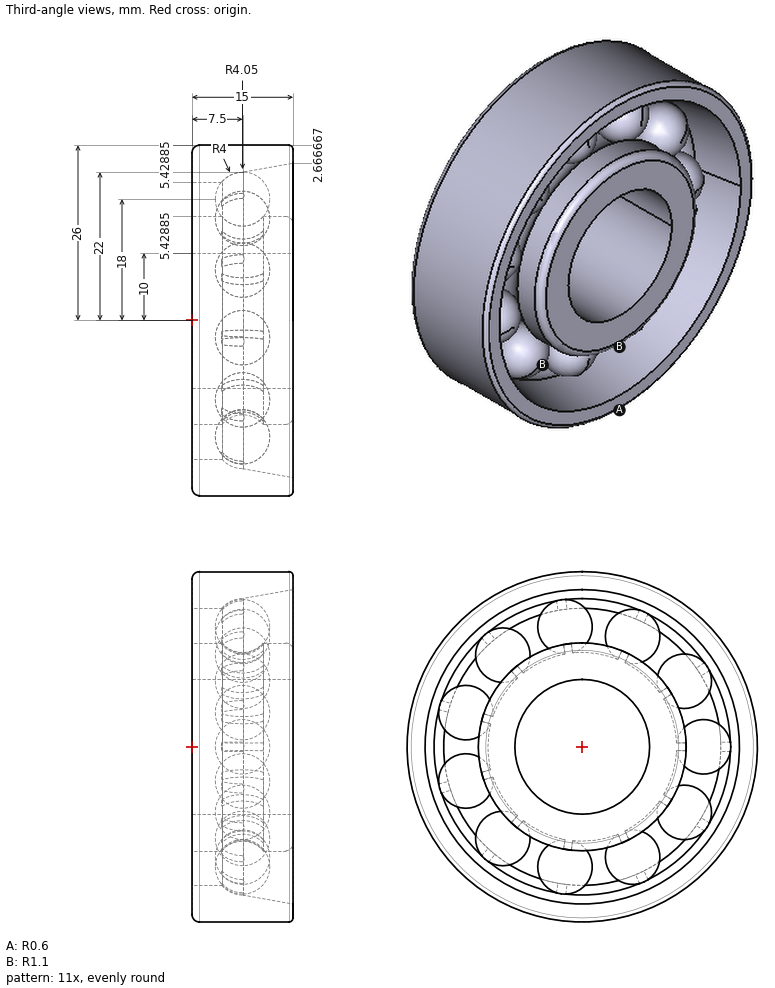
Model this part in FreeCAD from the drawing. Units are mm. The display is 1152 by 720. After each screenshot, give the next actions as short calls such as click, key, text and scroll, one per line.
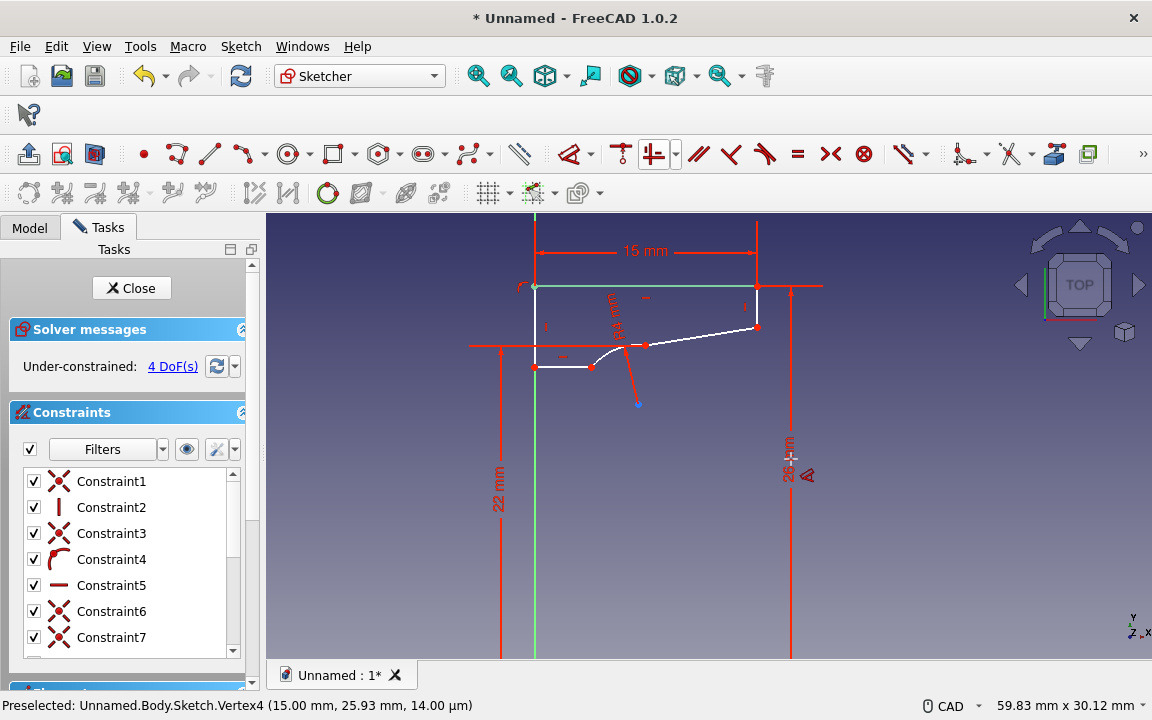
click(646, 346)
click(552, 312)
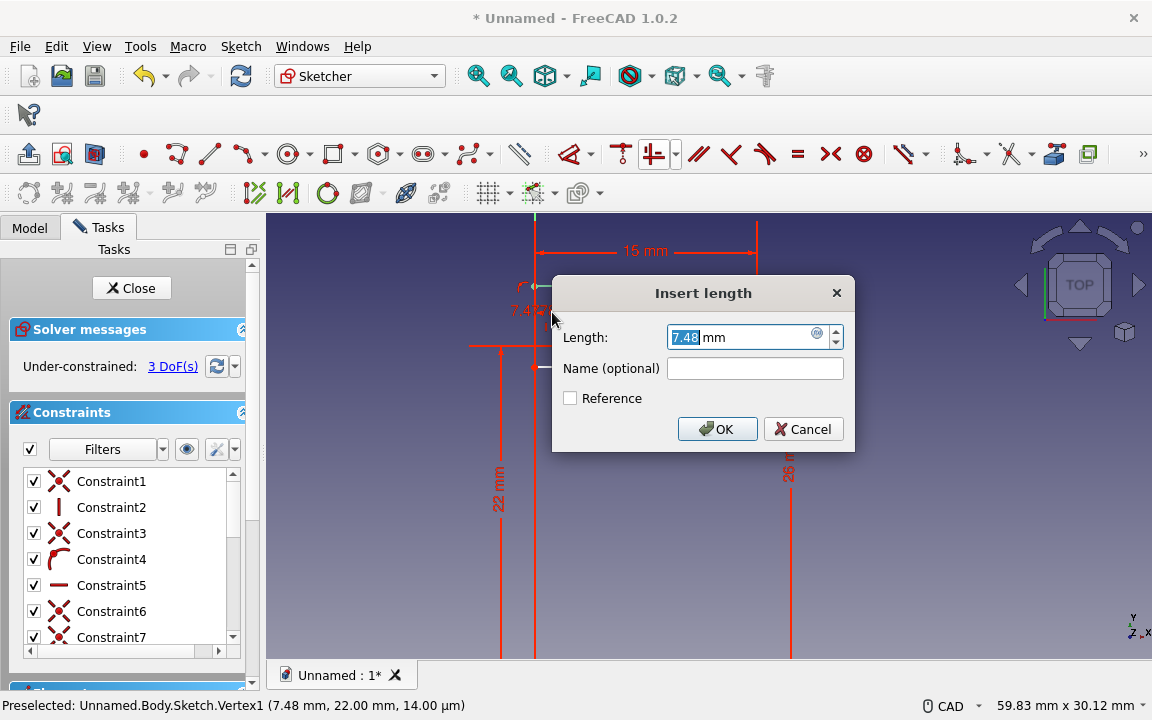
text(7.5)
key(Return)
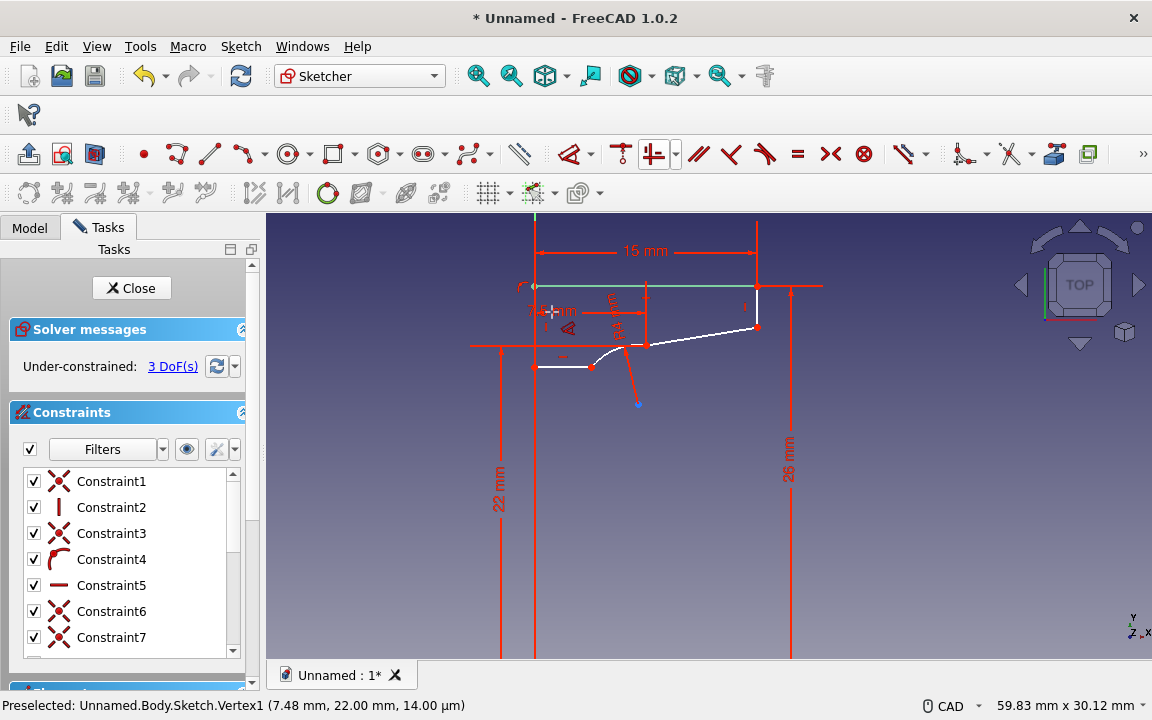
click(638, 404)
click(610, 370)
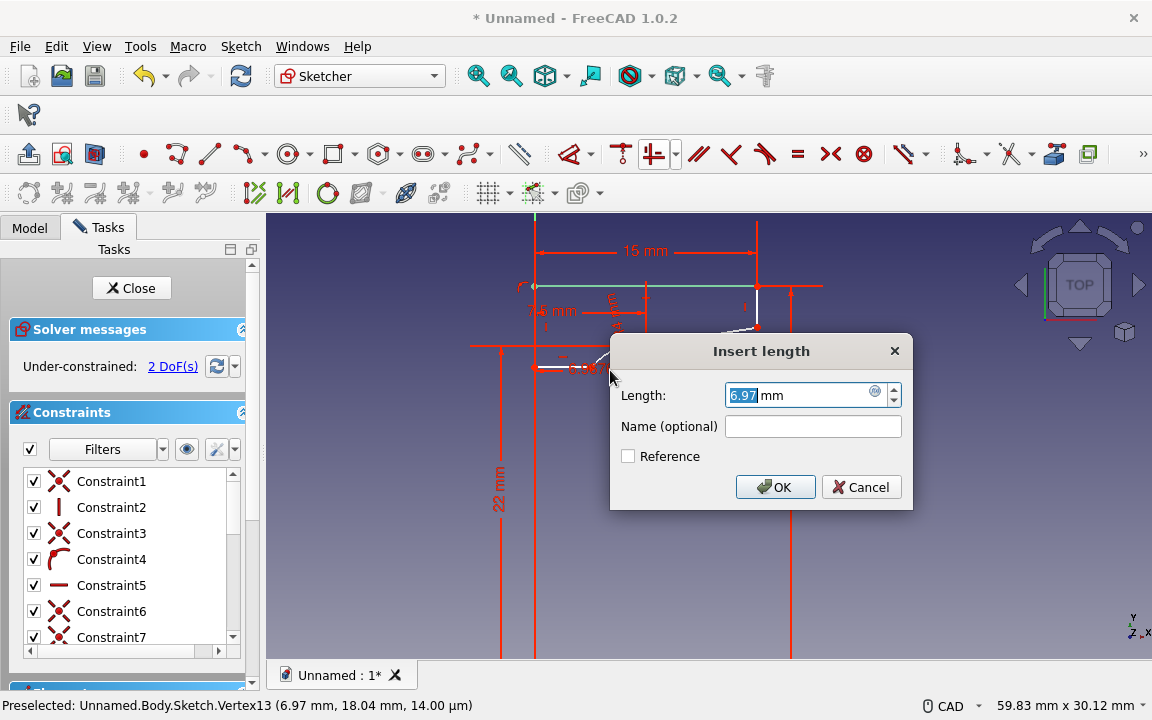
text(7.5)
key(Return)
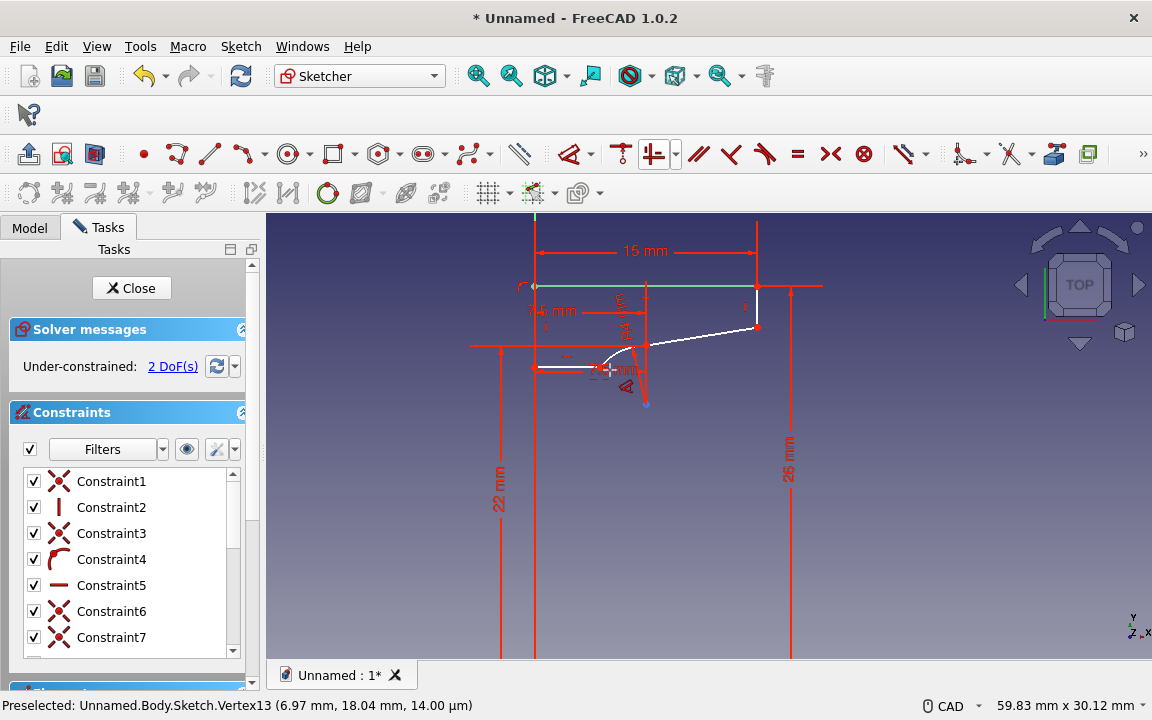
click(535, 311)
click(501, 345)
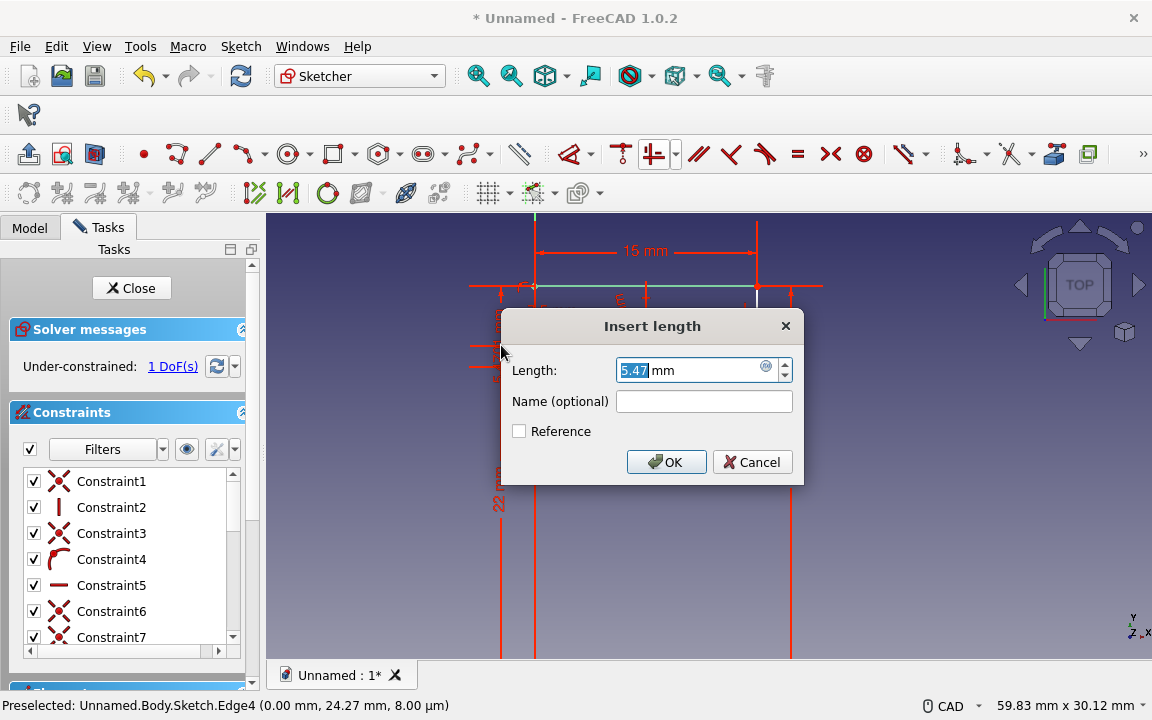
text(5.42885)
key(Return)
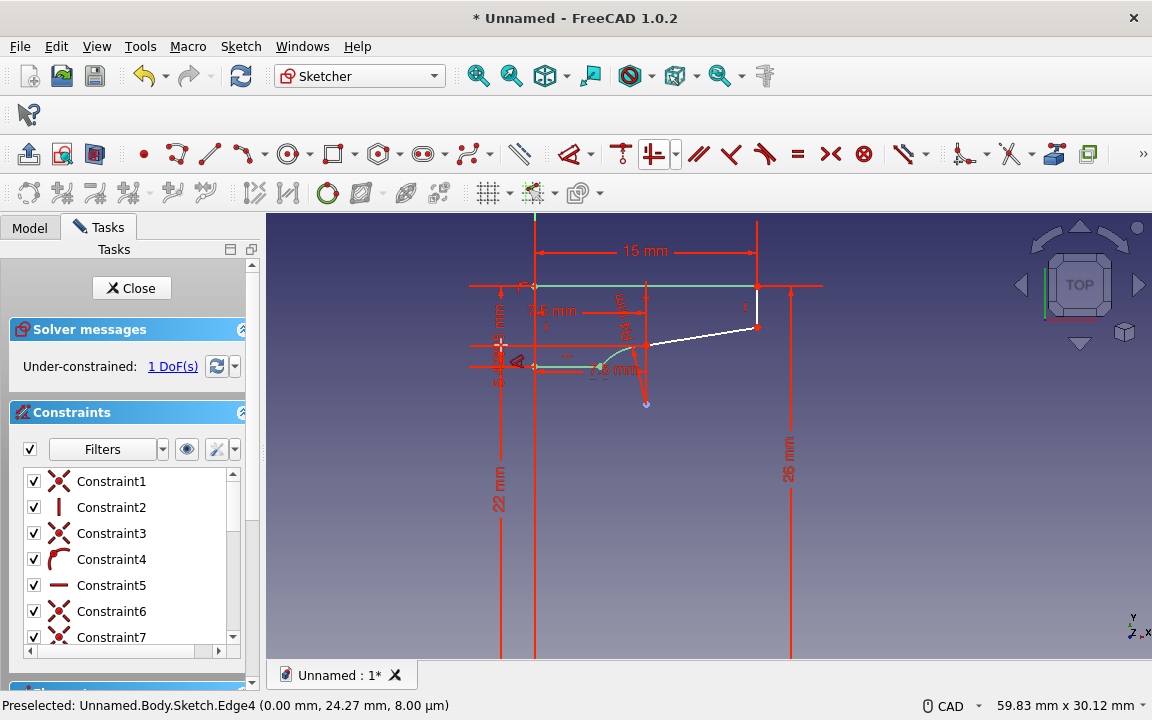
click(757, 315)
click(791, 307)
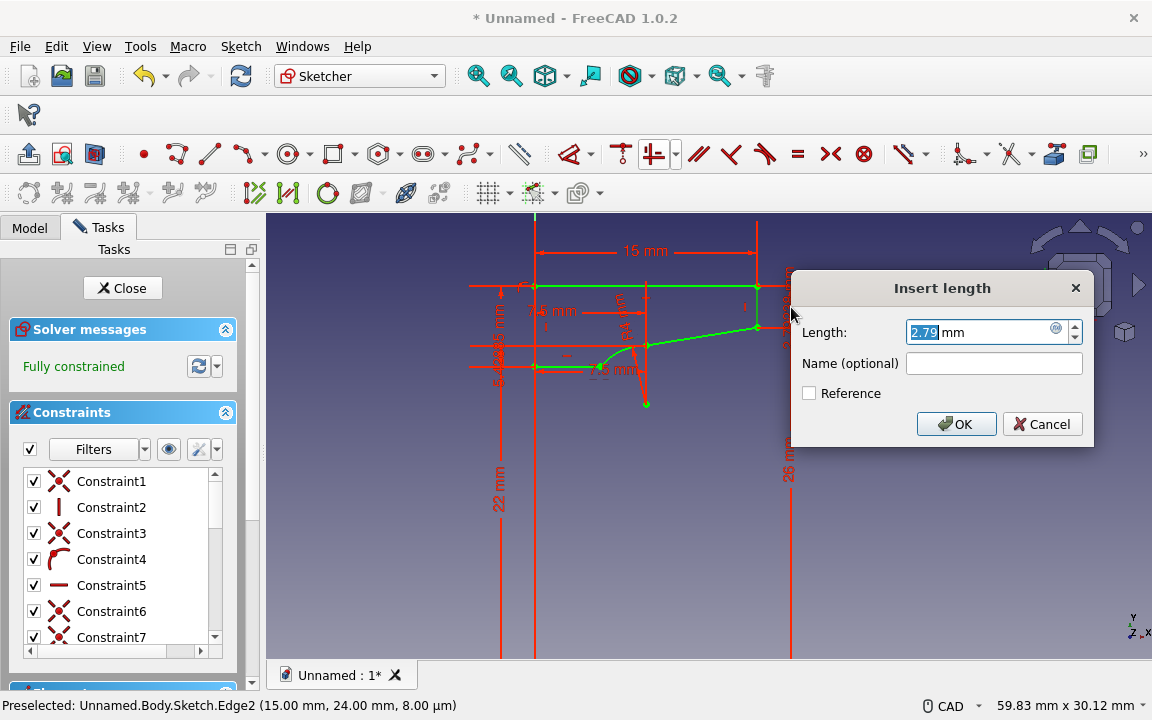
text(2.666667)
key(Return)
key(Escape)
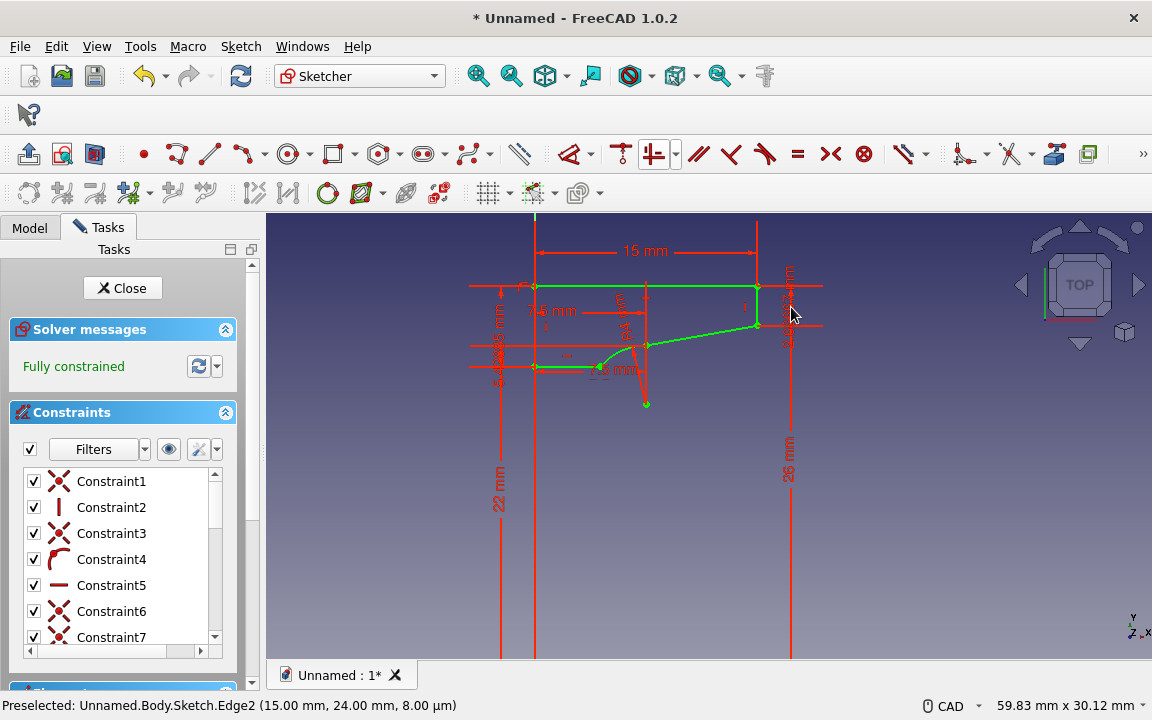
click(123, 288)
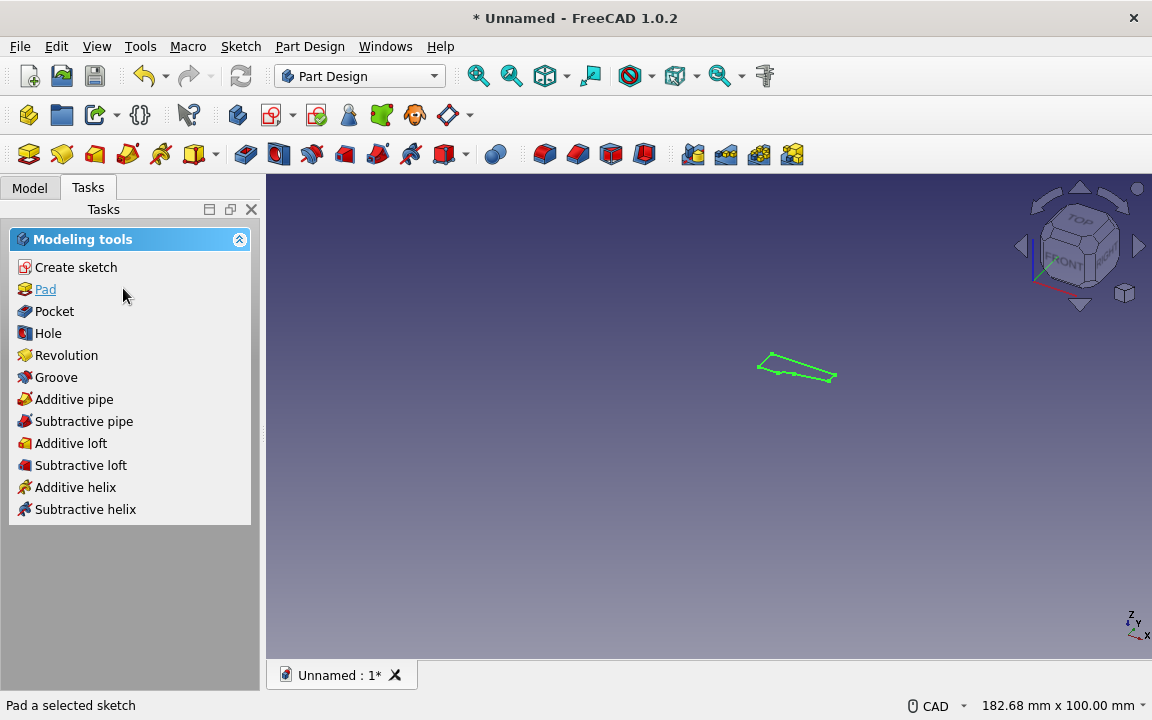
click(62, 154)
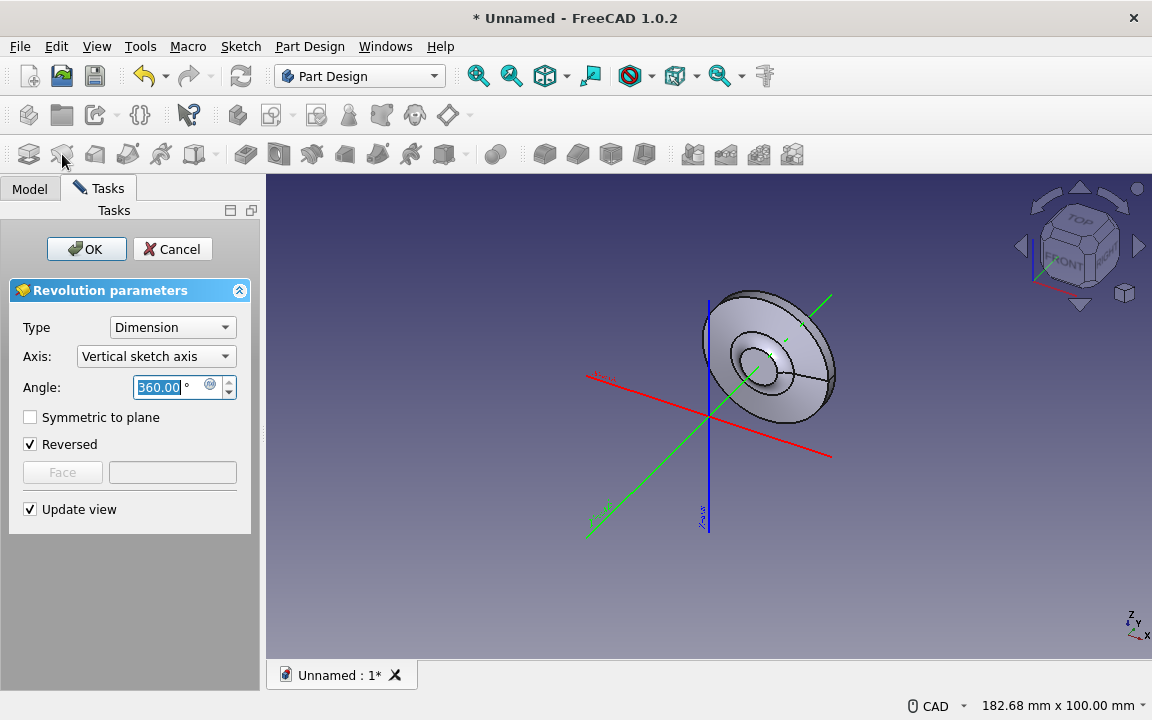
click(157, 356)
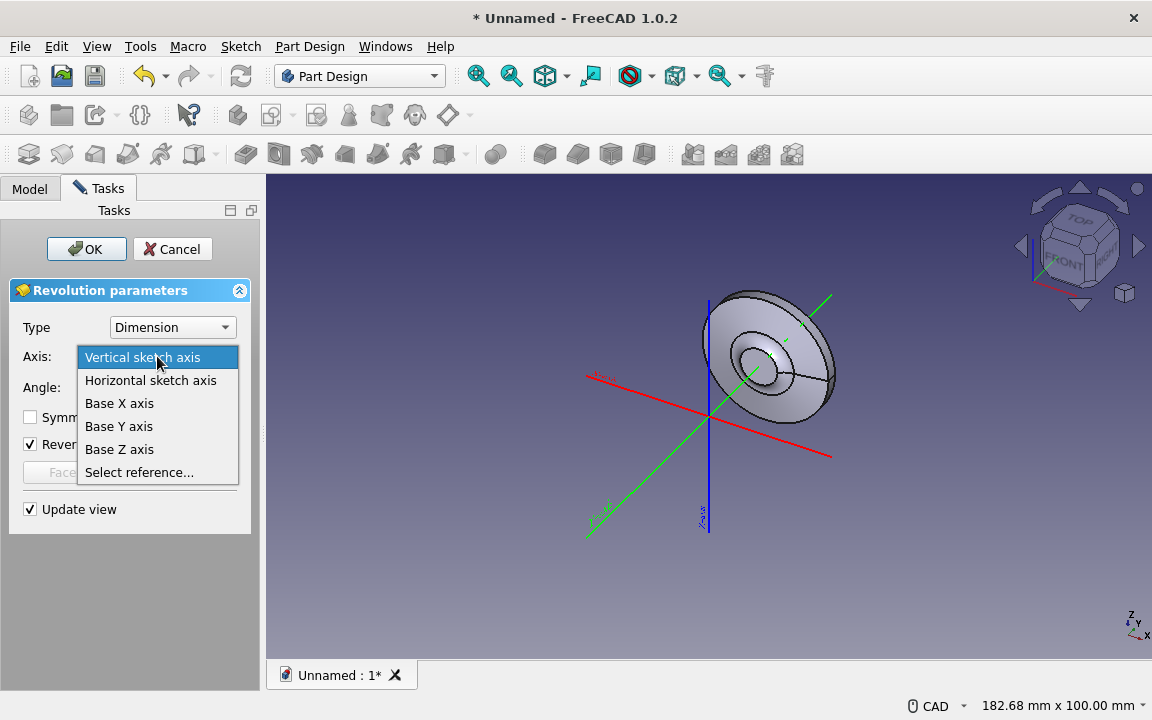
click(156, 380)